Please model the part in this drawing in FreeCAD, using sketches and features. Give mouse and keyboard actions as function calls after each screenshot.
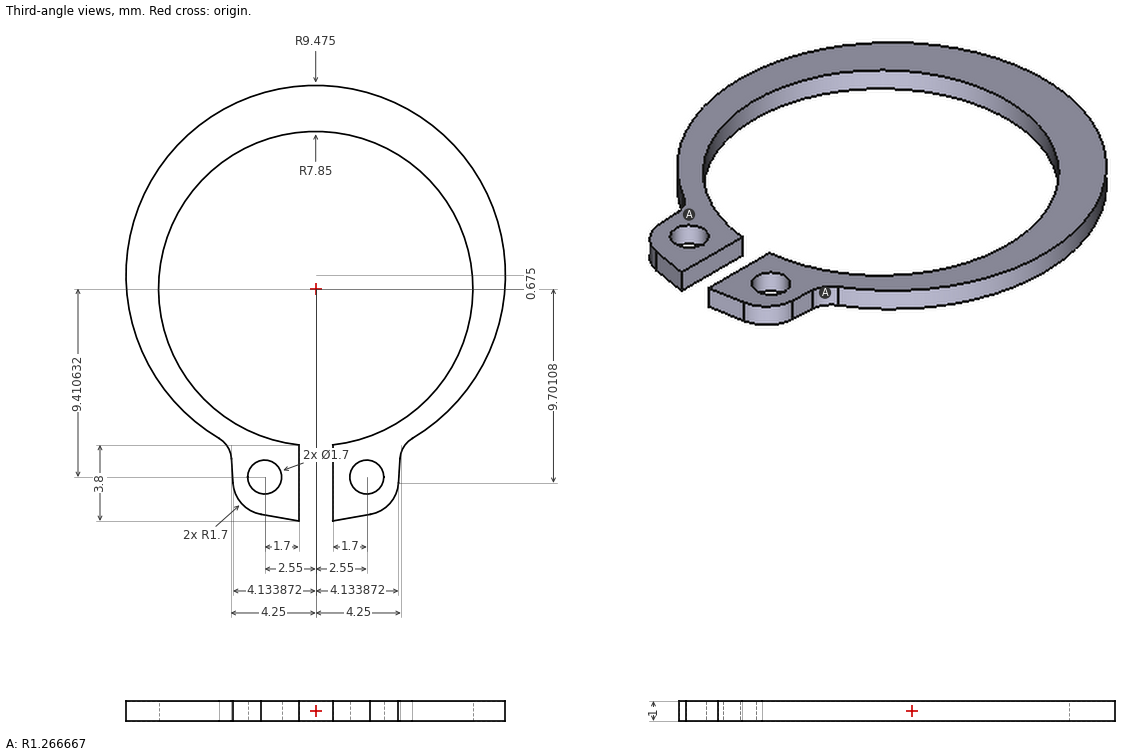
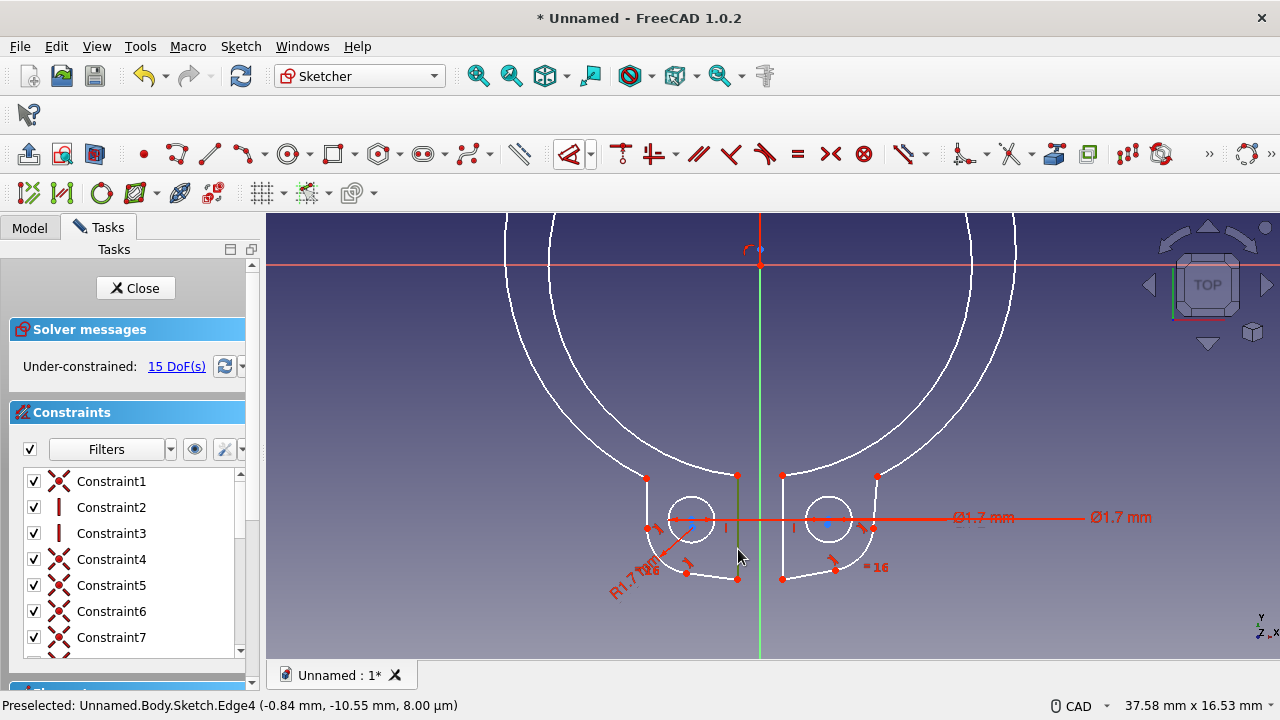
key(i)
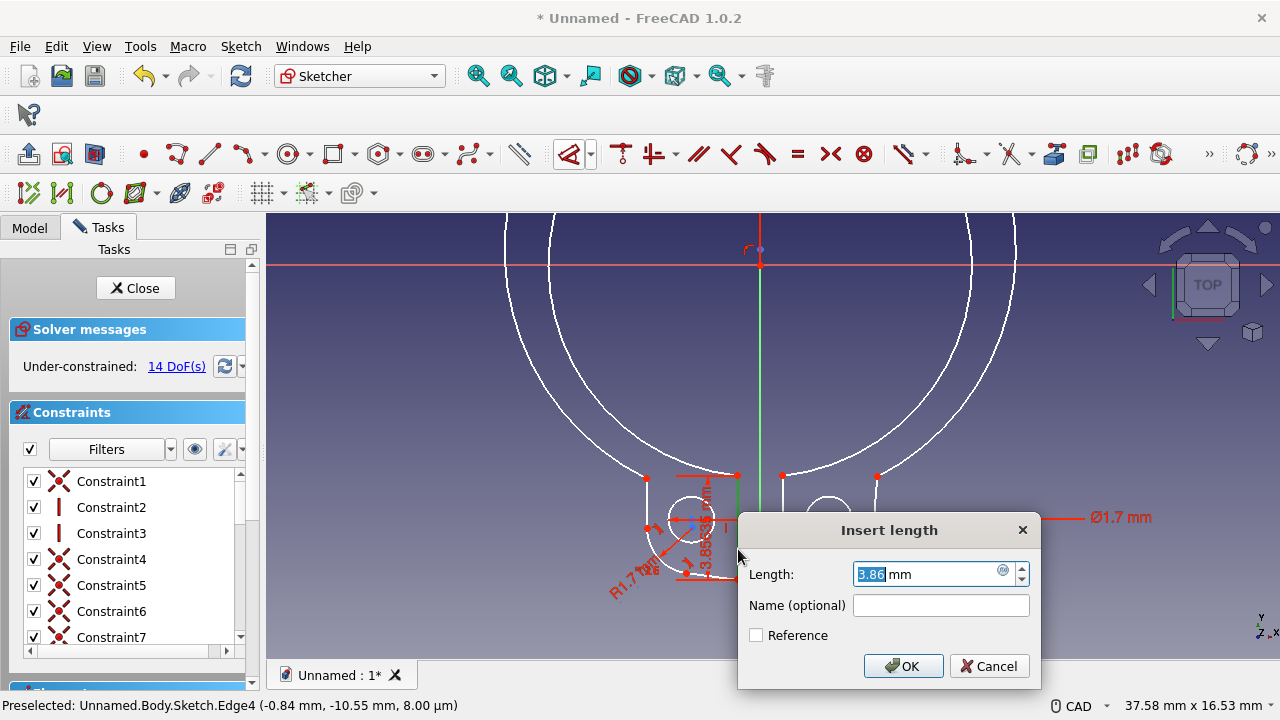
text(3.8)
key(Return)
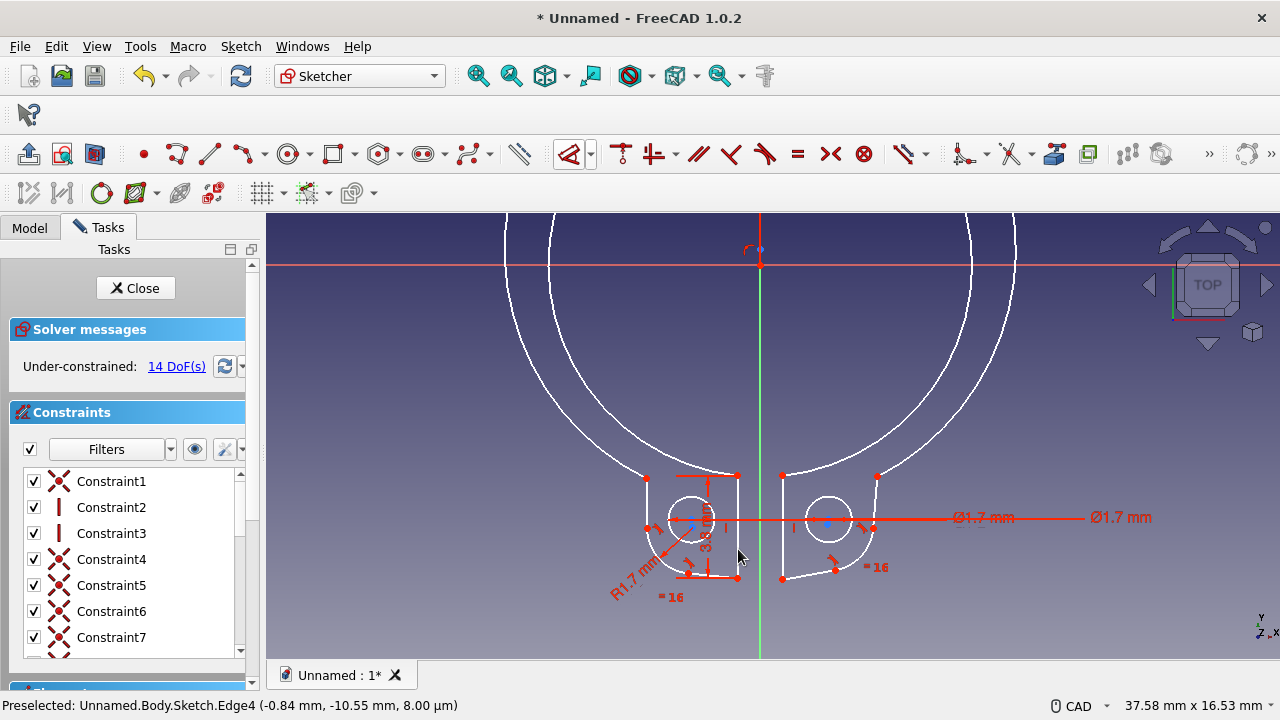
click(783, 507)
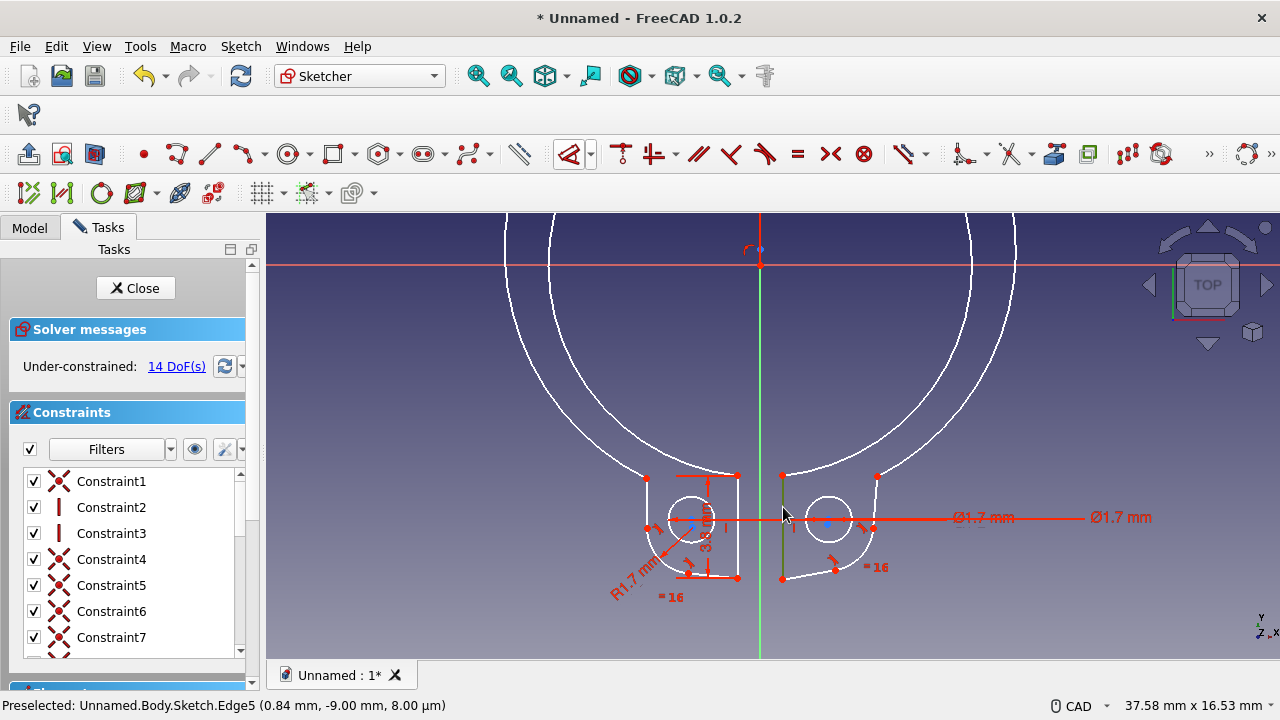
key(i)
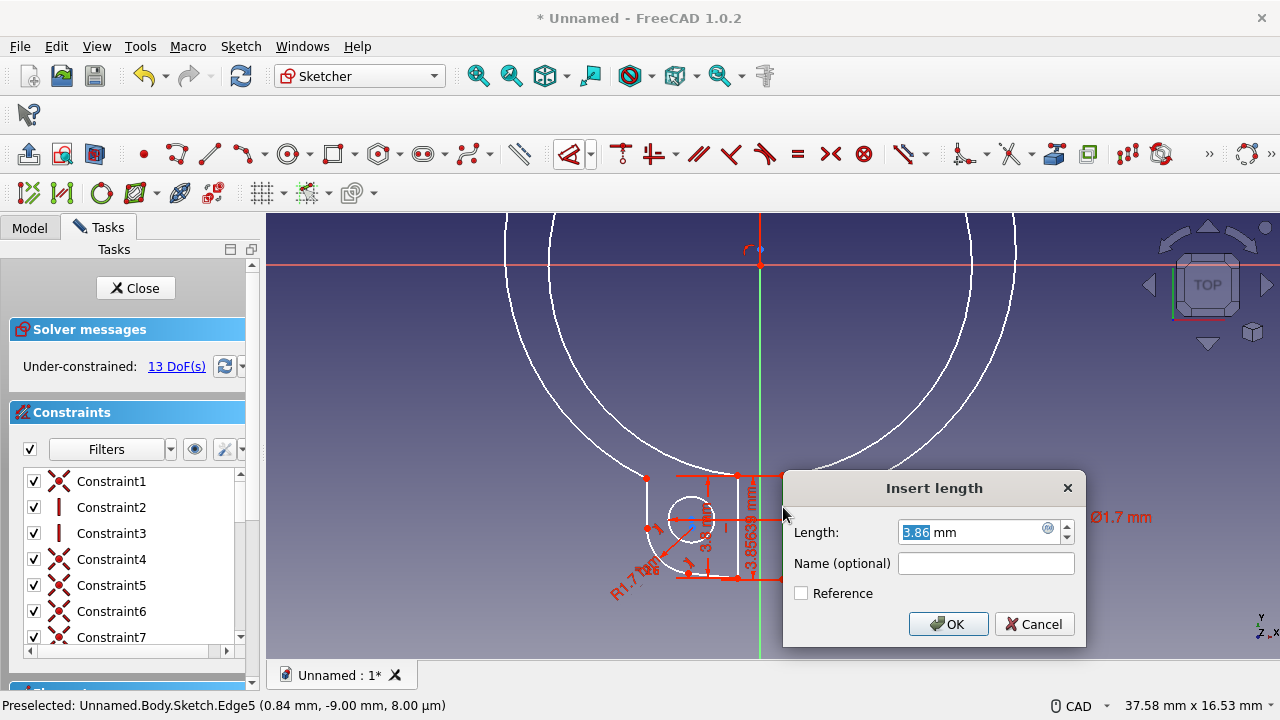
text(3.8)
key(Return)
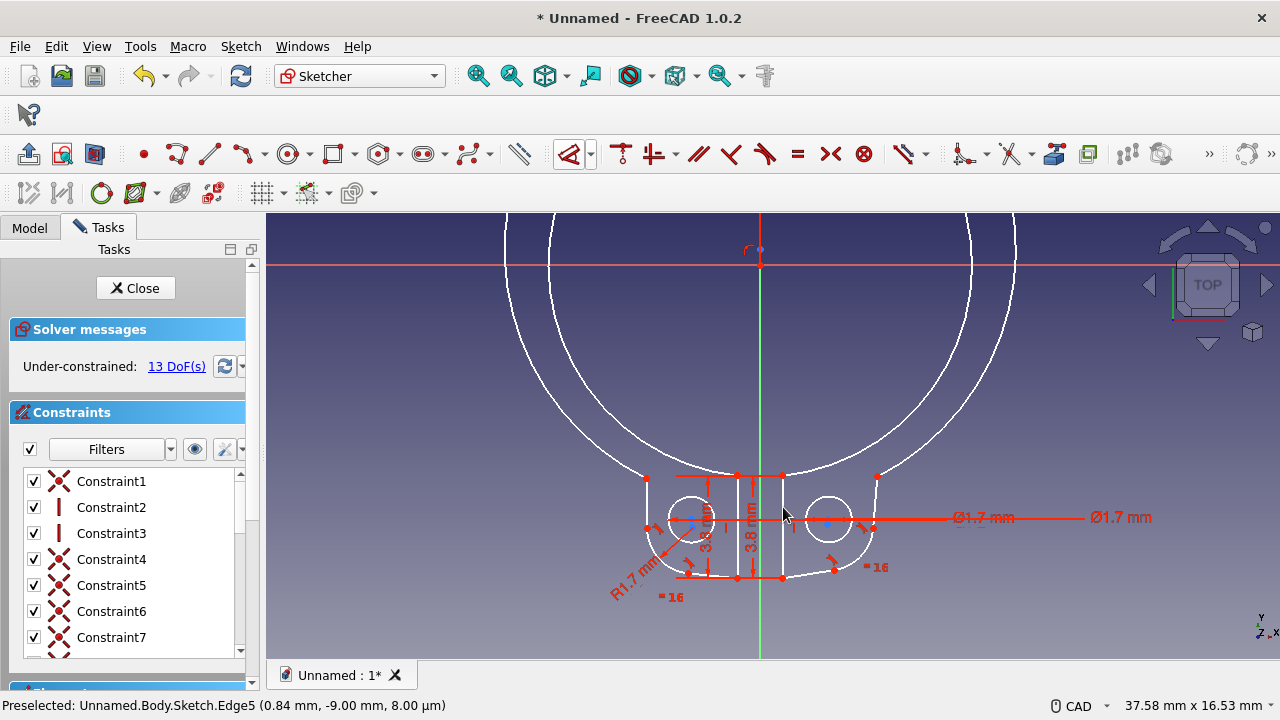
scroll(691, 520, up, 2)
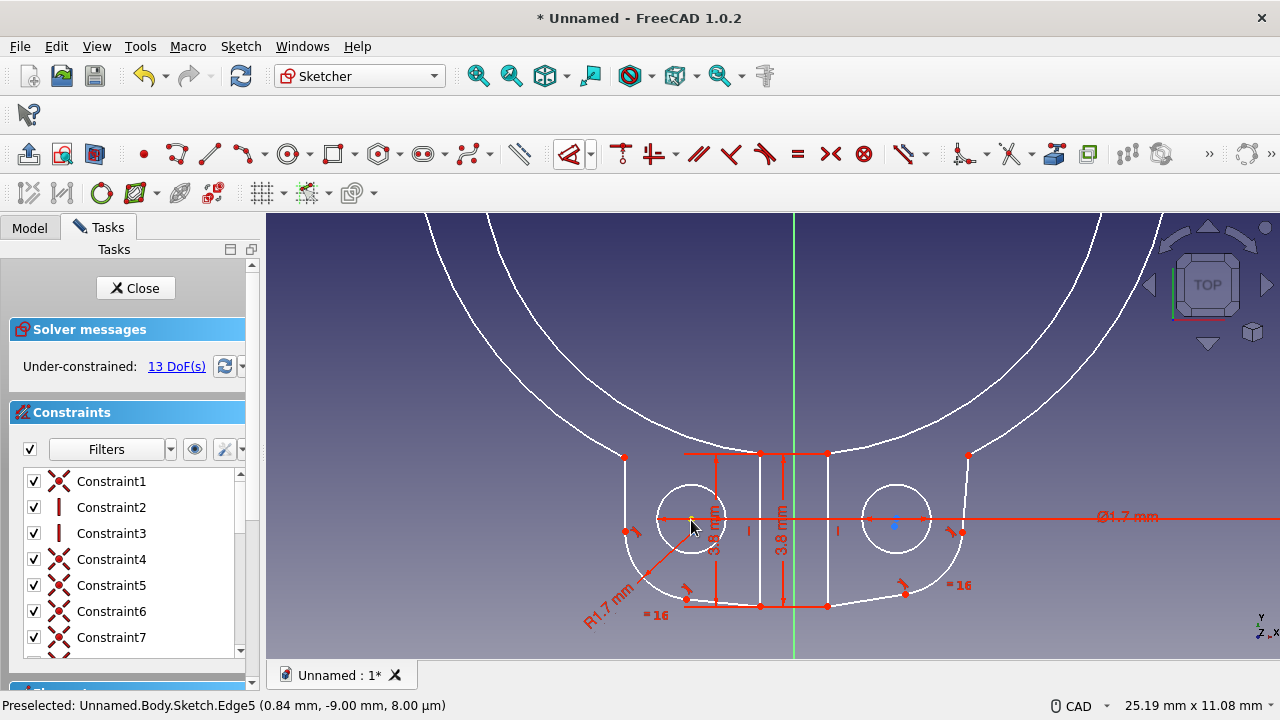
click(691, 519)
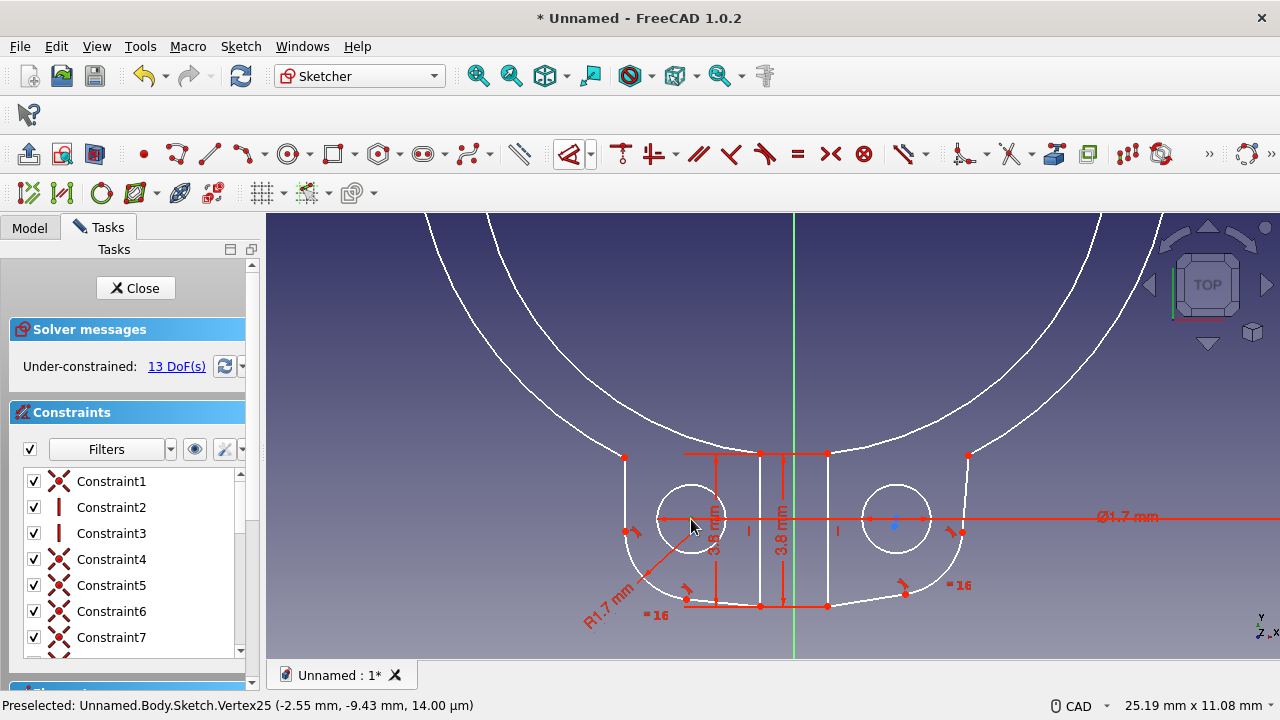
key(l)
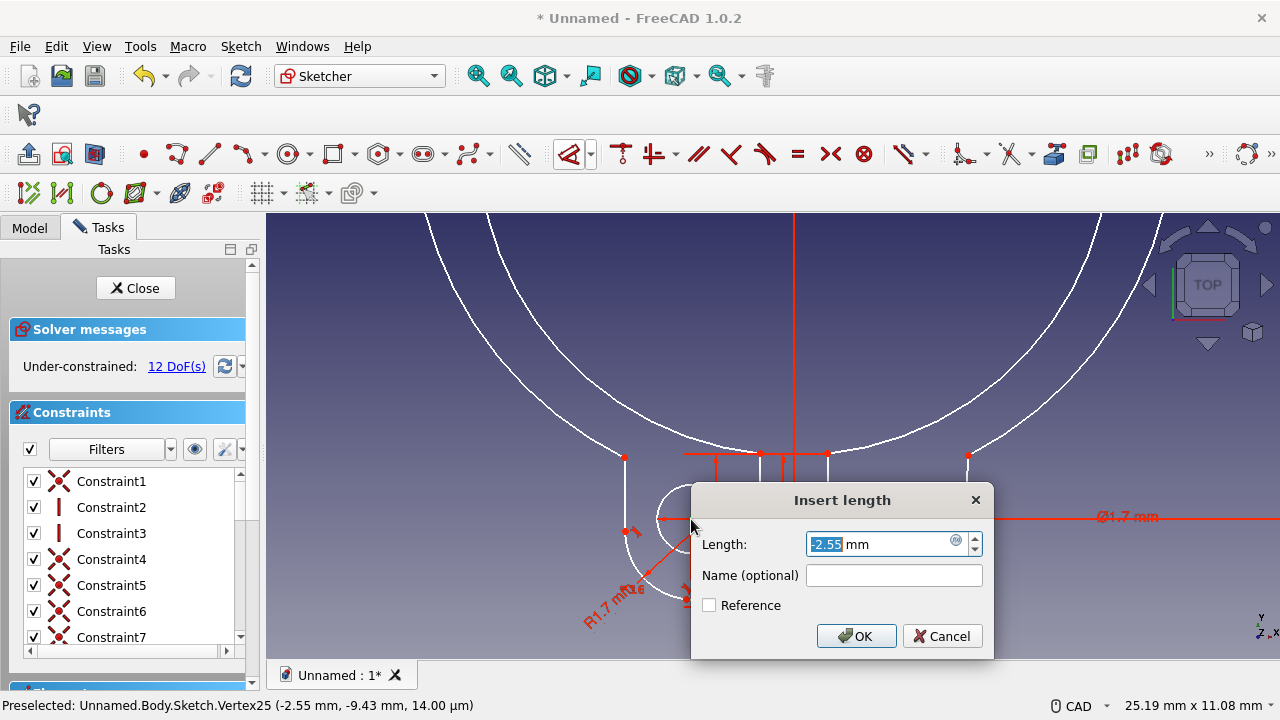
text(-2.55)
key(Return)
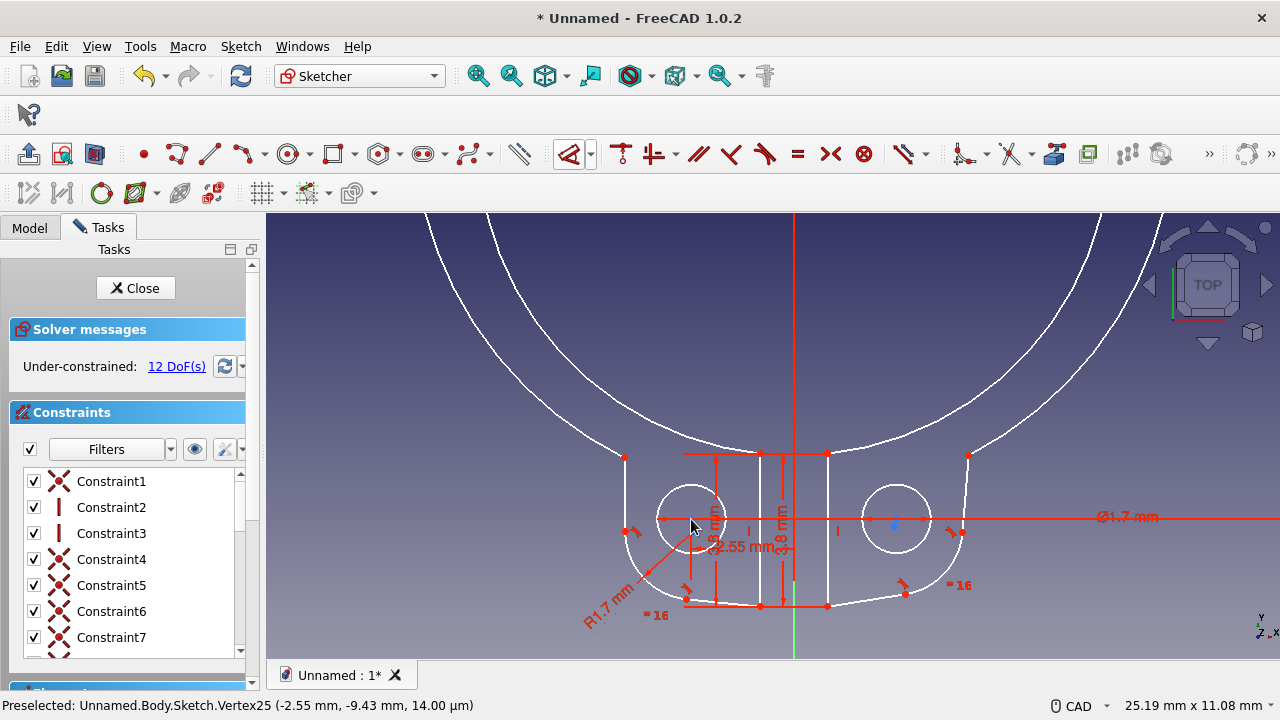
scroll(897, 519, up, 3)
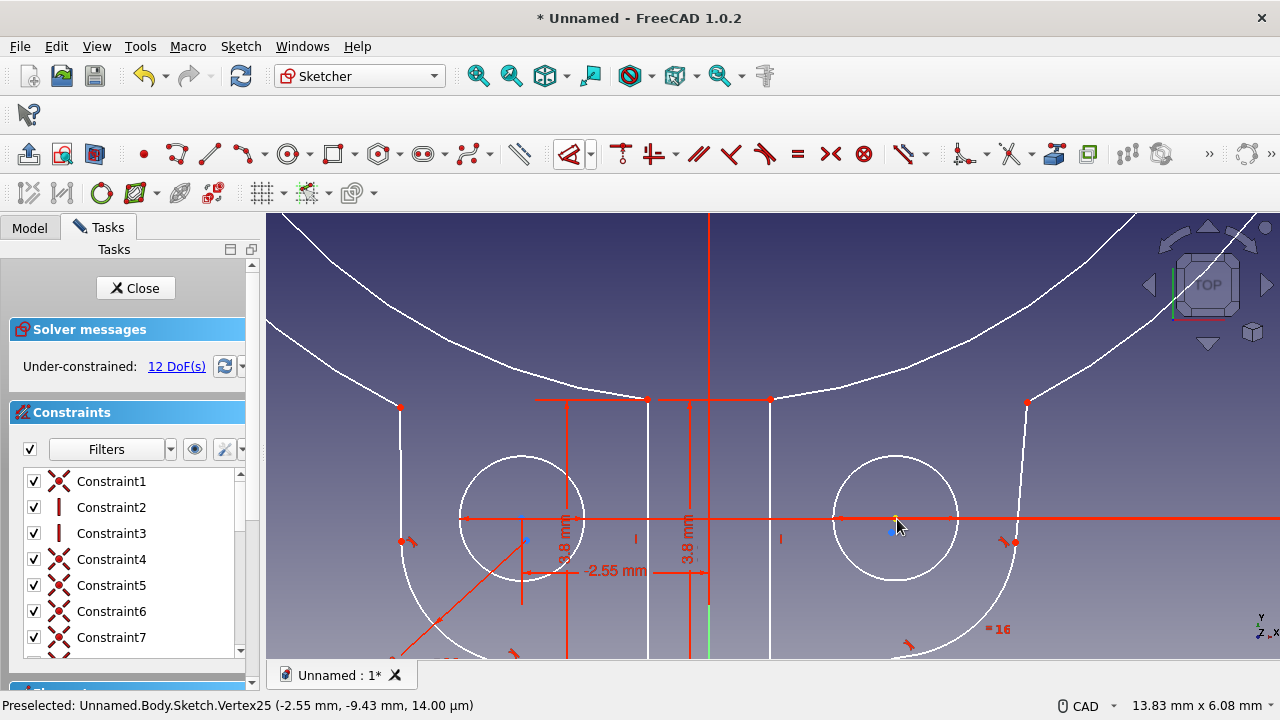
click(896, 518)